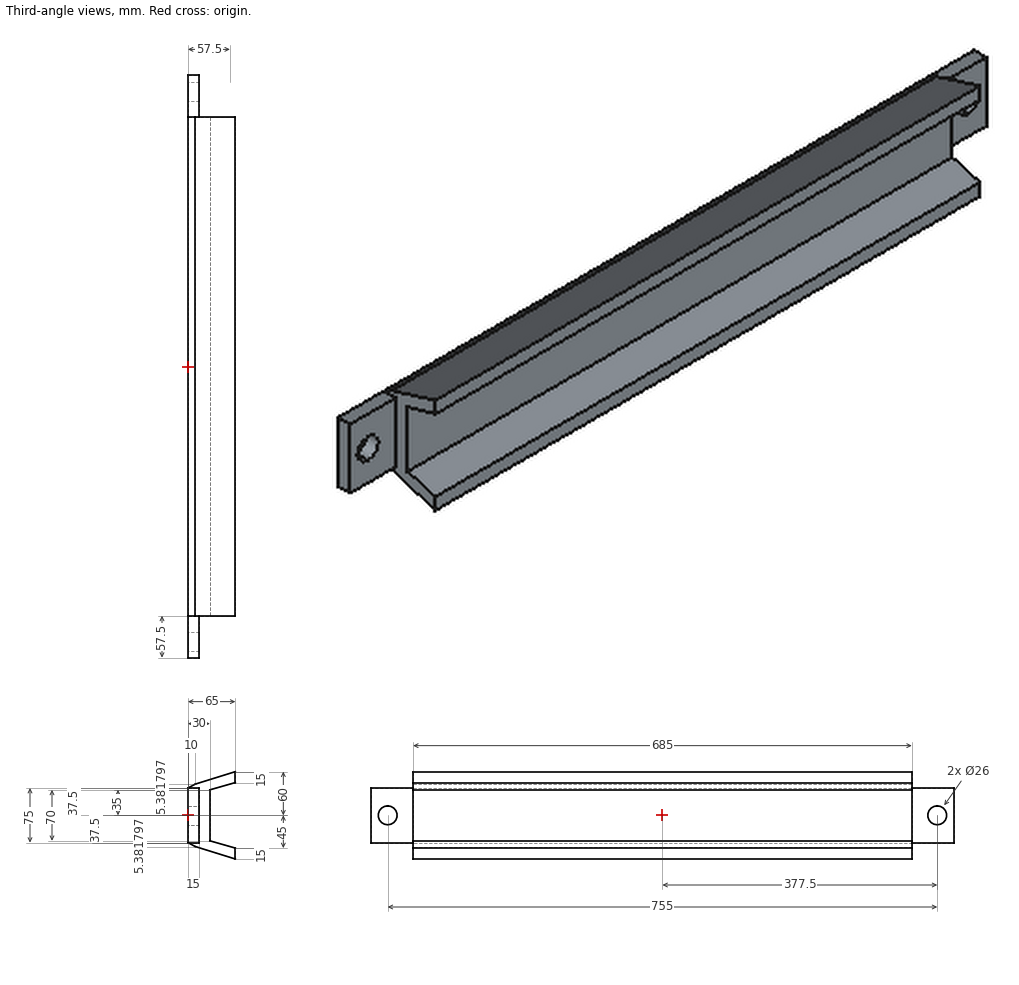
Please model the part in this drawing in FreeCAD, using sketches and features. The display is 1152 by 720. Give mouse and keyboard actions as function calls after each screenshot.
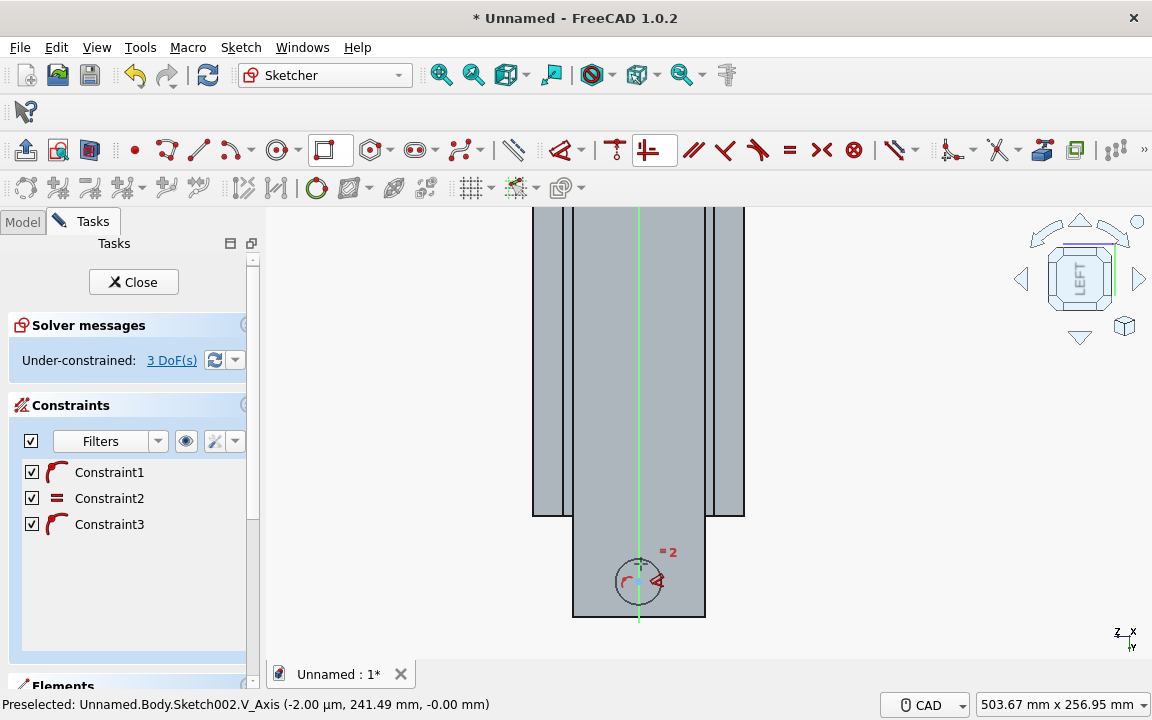
click(639, 559)
click(666, 534)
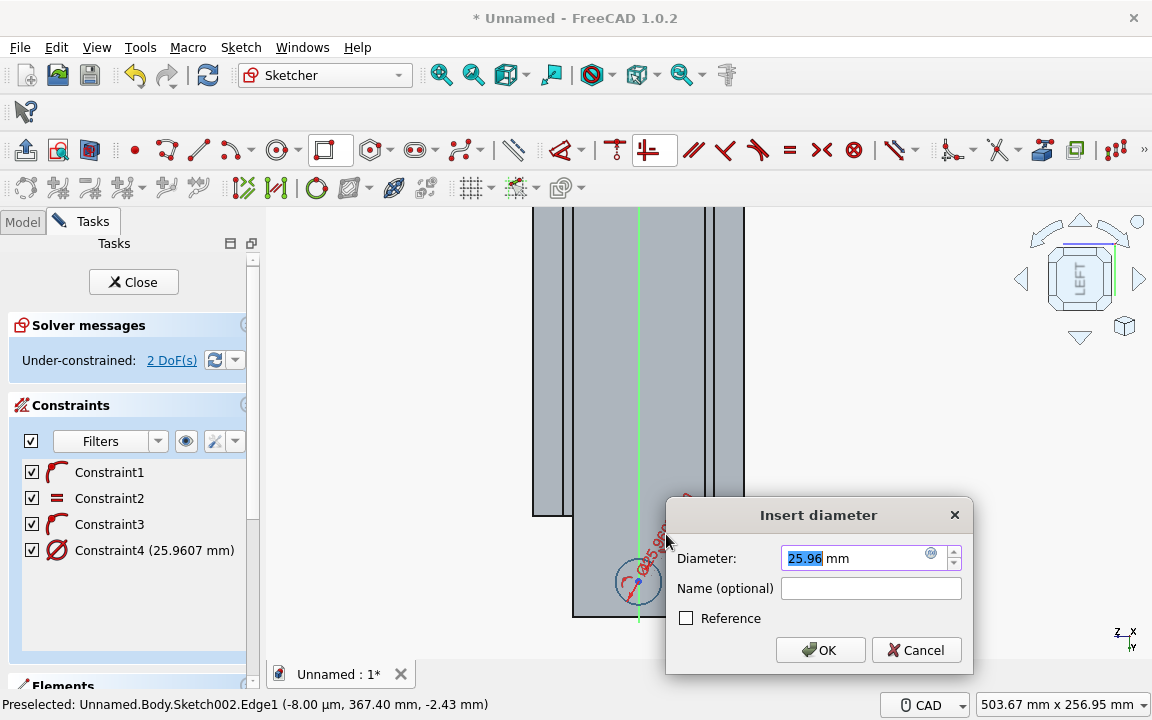
text(26)
key(Return)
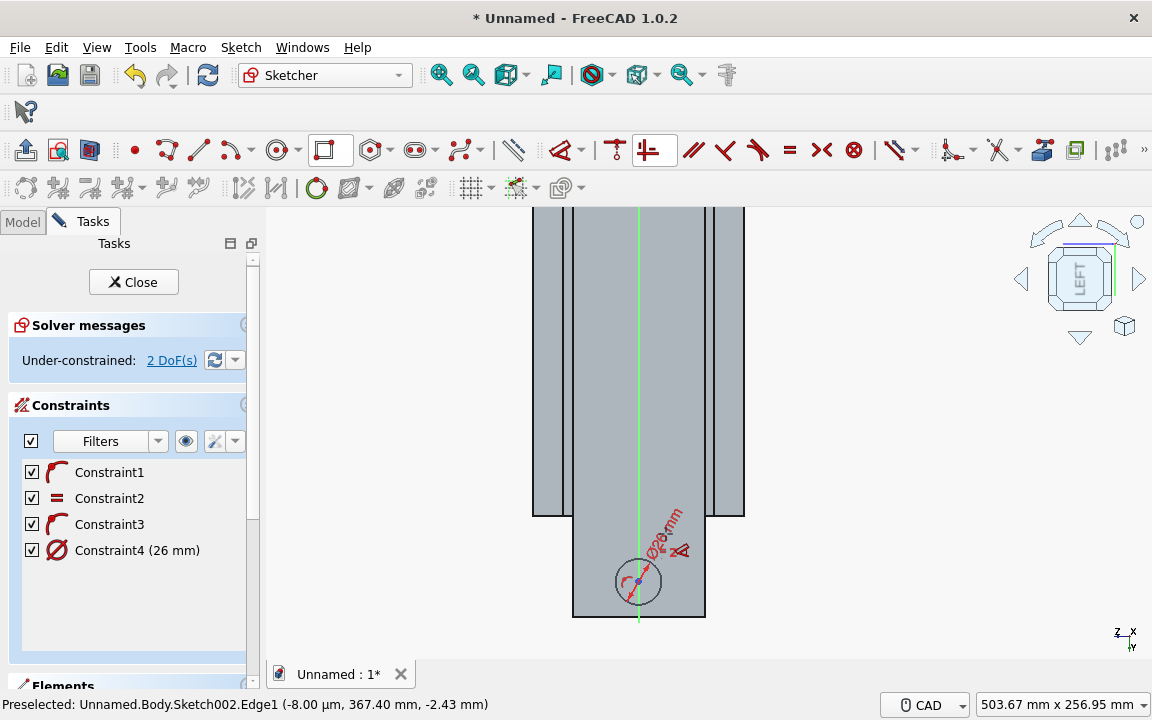
scroll(641, 564, down, 8)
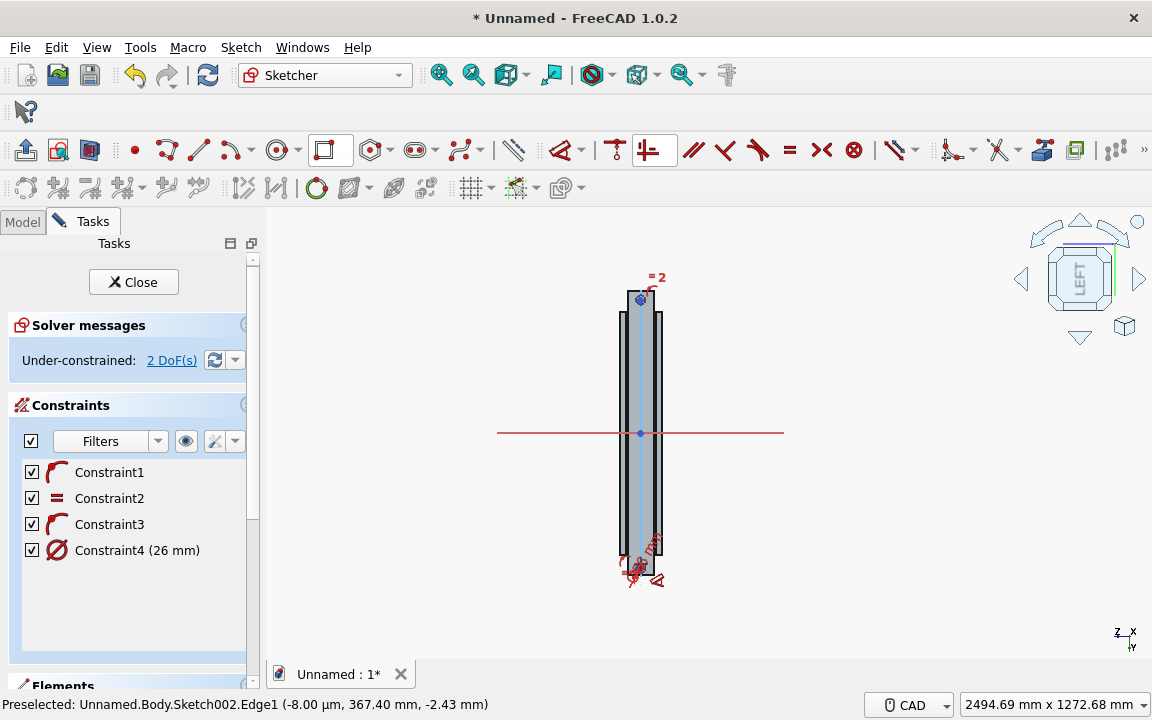
click(641, 568)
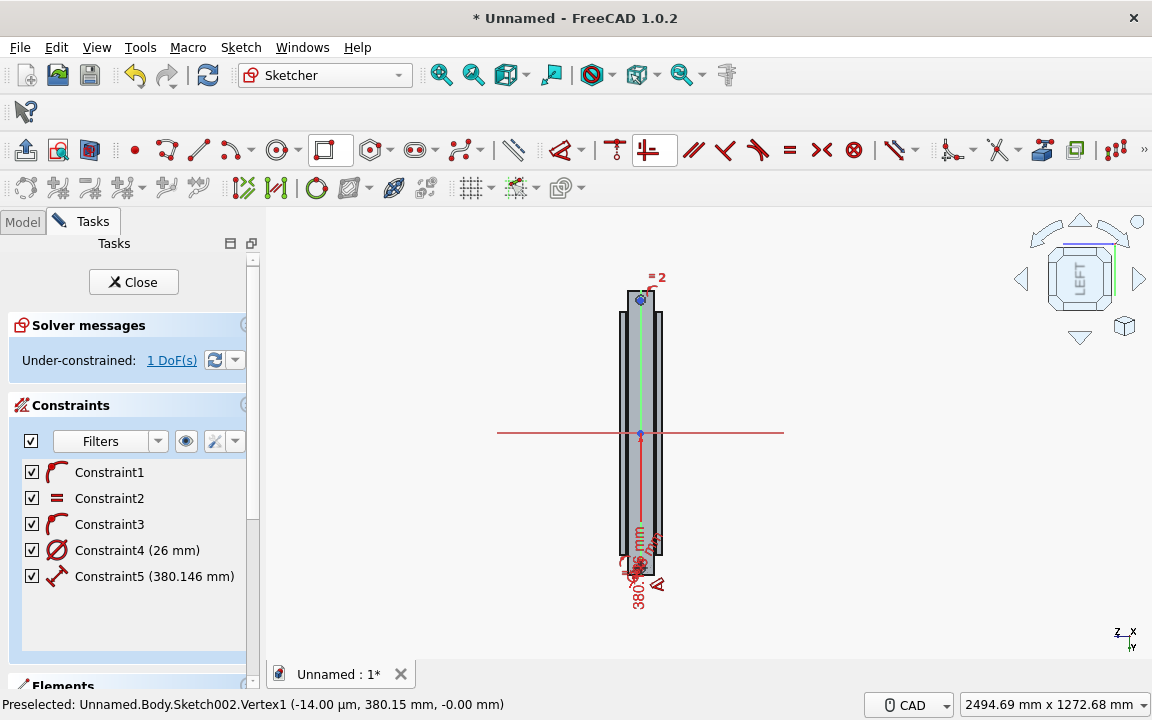
click(641, 300)
click(675, 372)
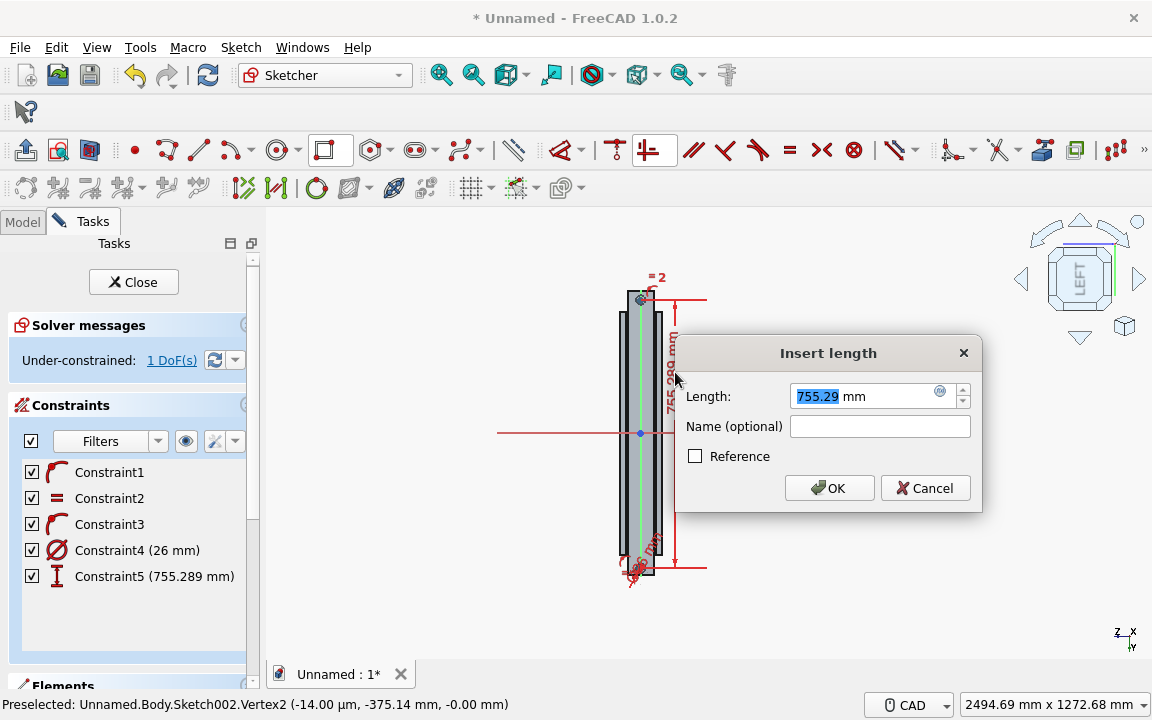
text(755)
key(Return)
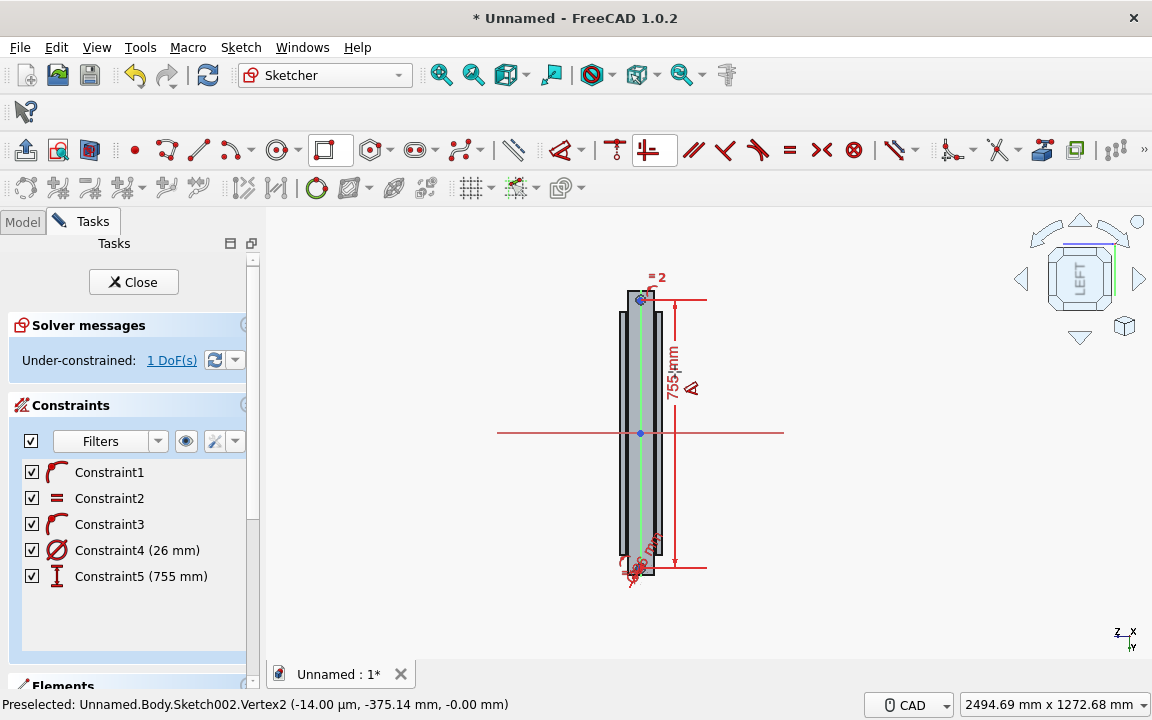
click(641, 568)
click(675, 501)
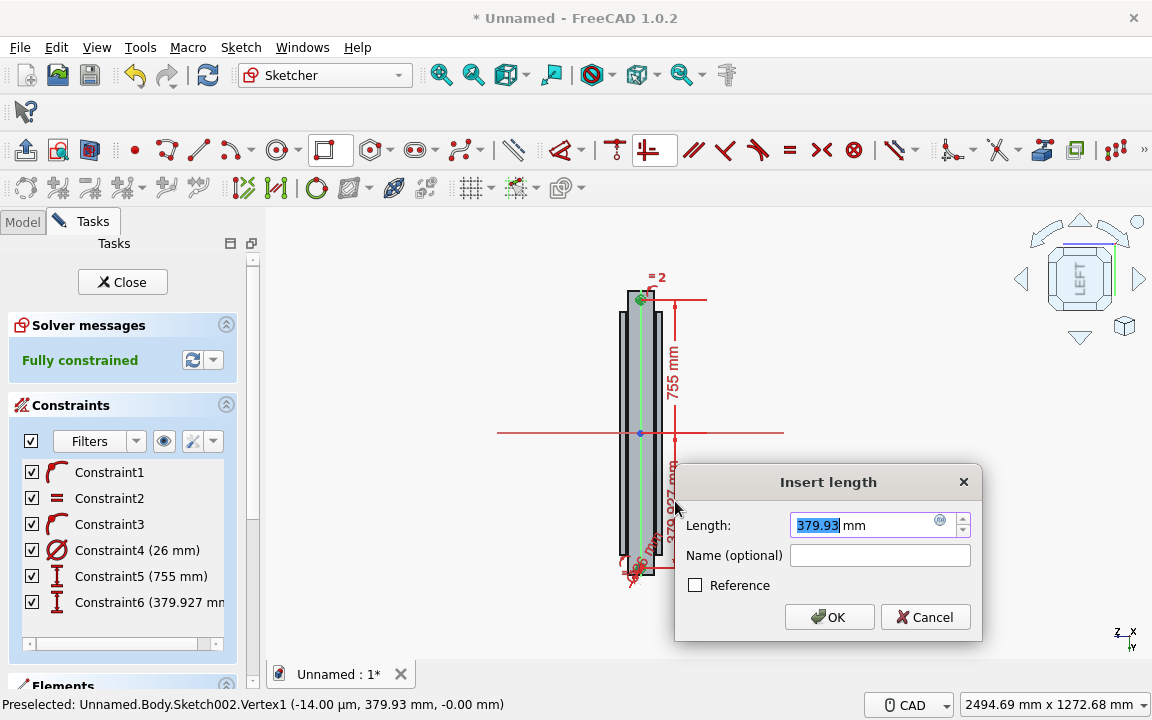
text(377.5)
key(Return)
key(Escape)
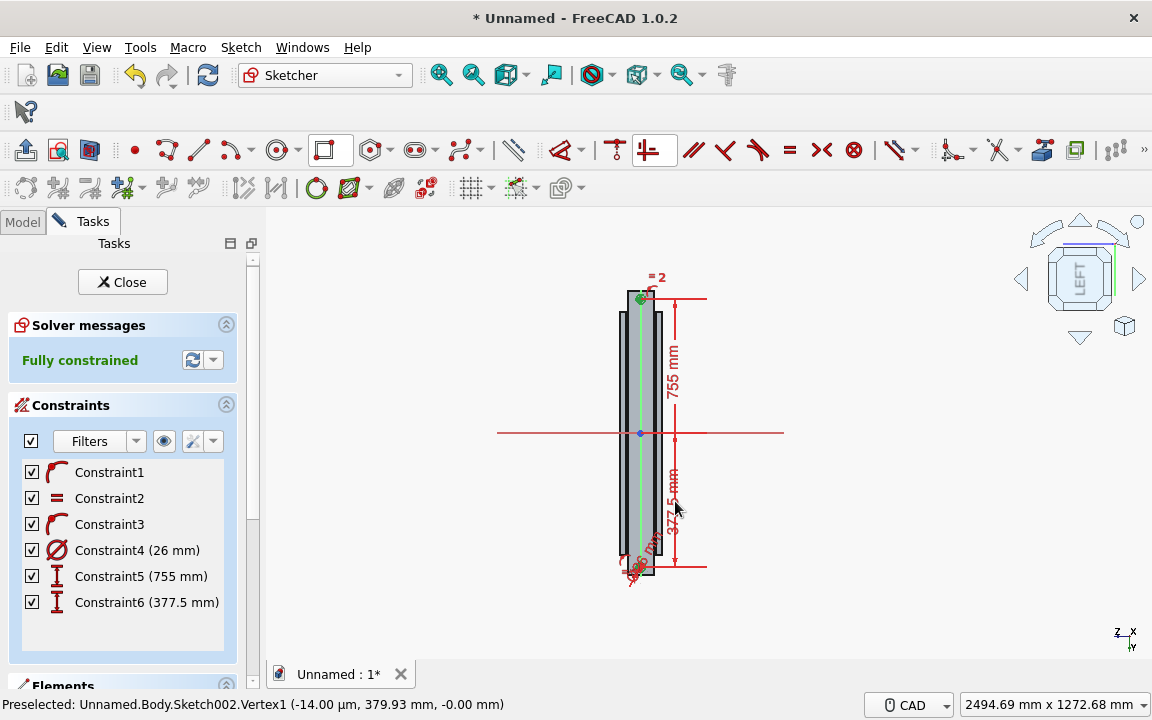
click(123, 282)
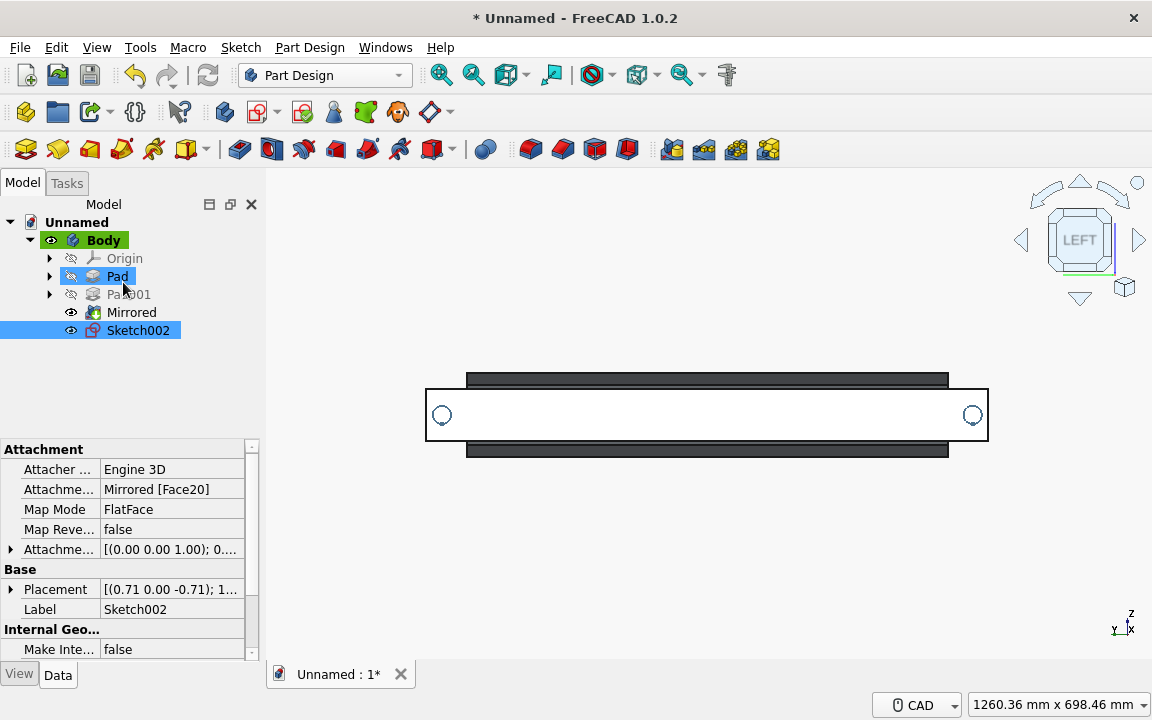
click(240, 150)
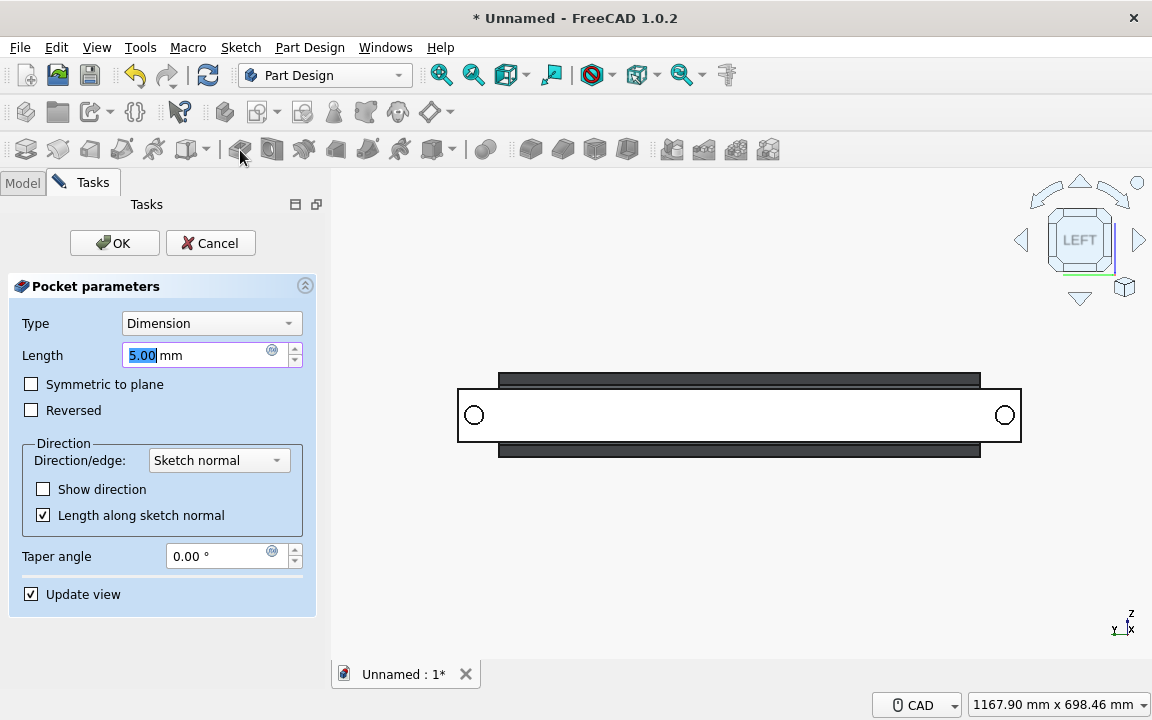
text(57.5)
key(Tab)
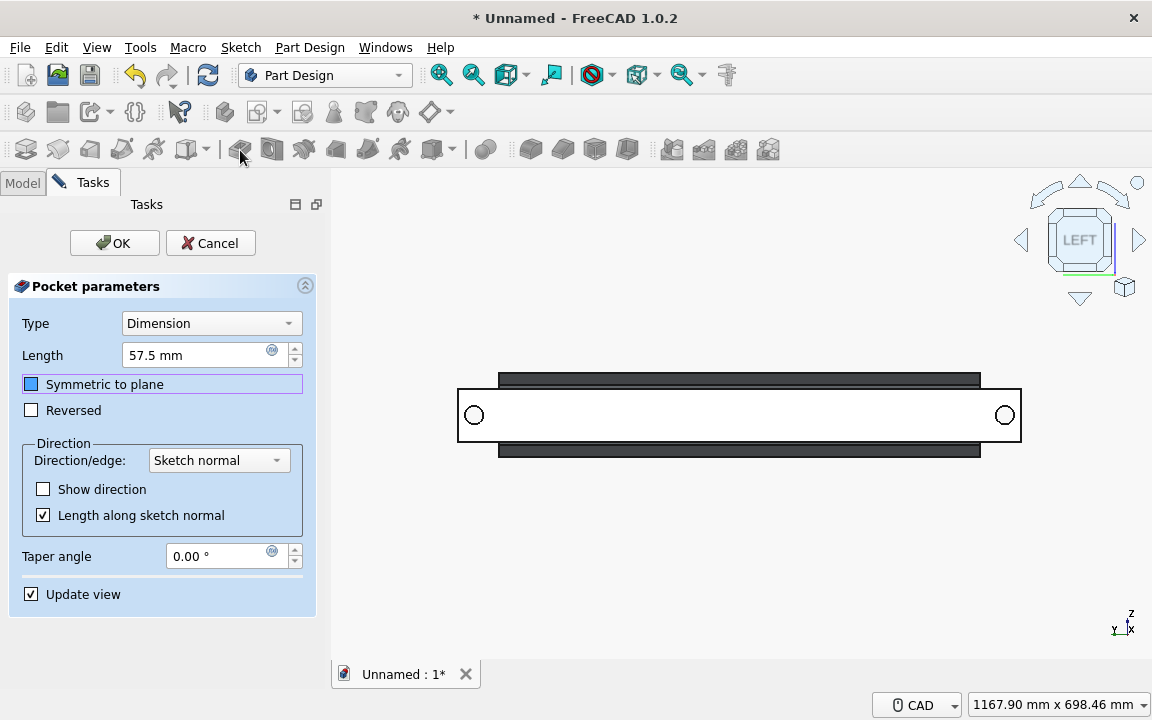
click(115, 243)